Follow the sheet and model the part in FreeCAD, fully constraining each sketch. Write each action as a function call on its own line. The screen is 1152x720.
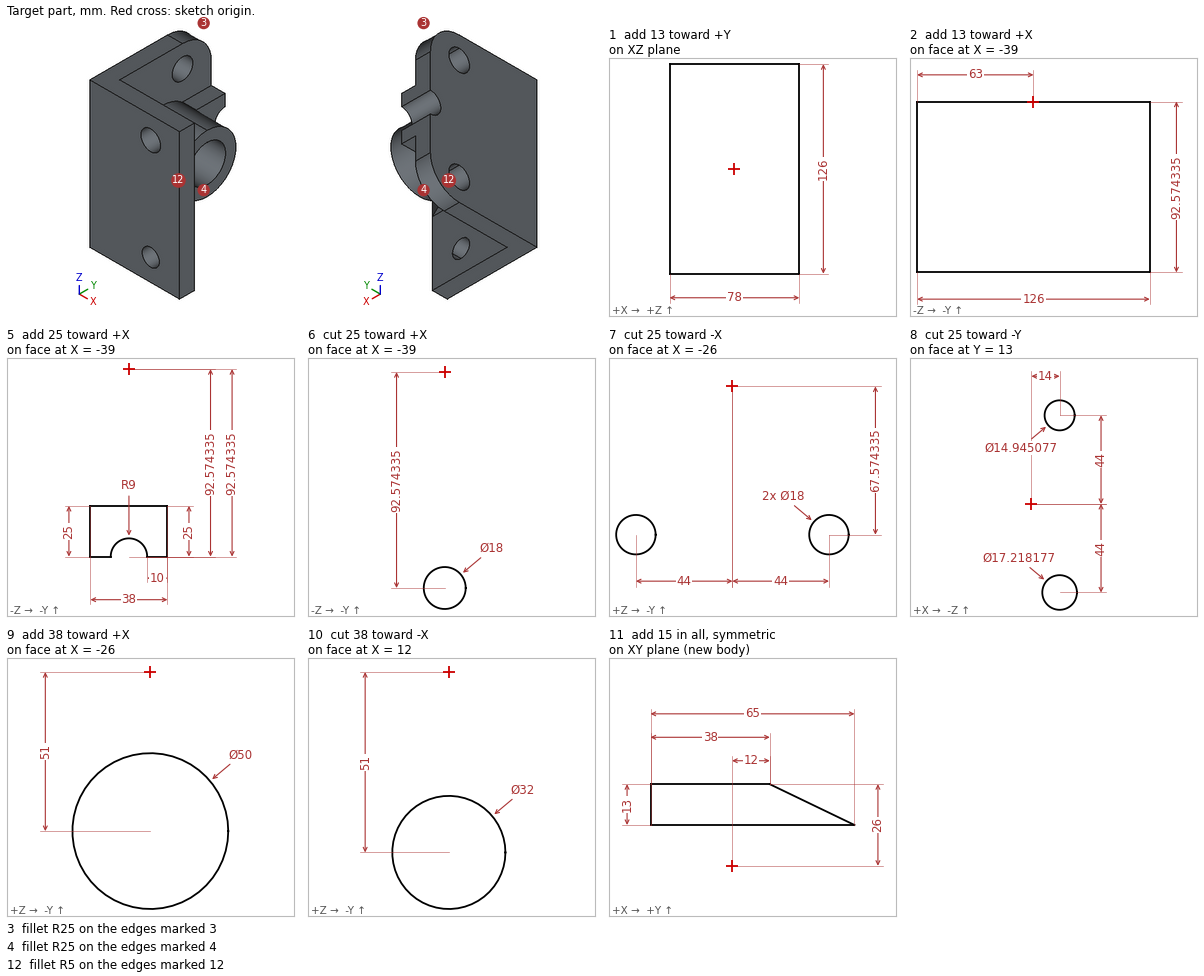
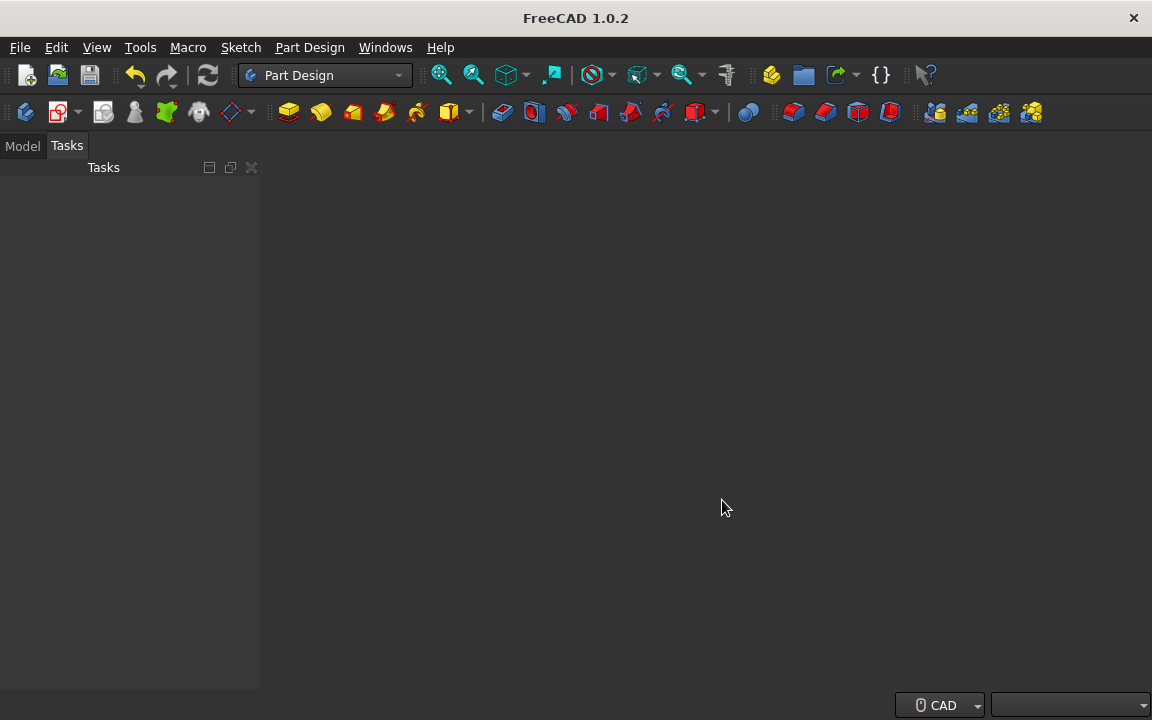
key(ctrl+n)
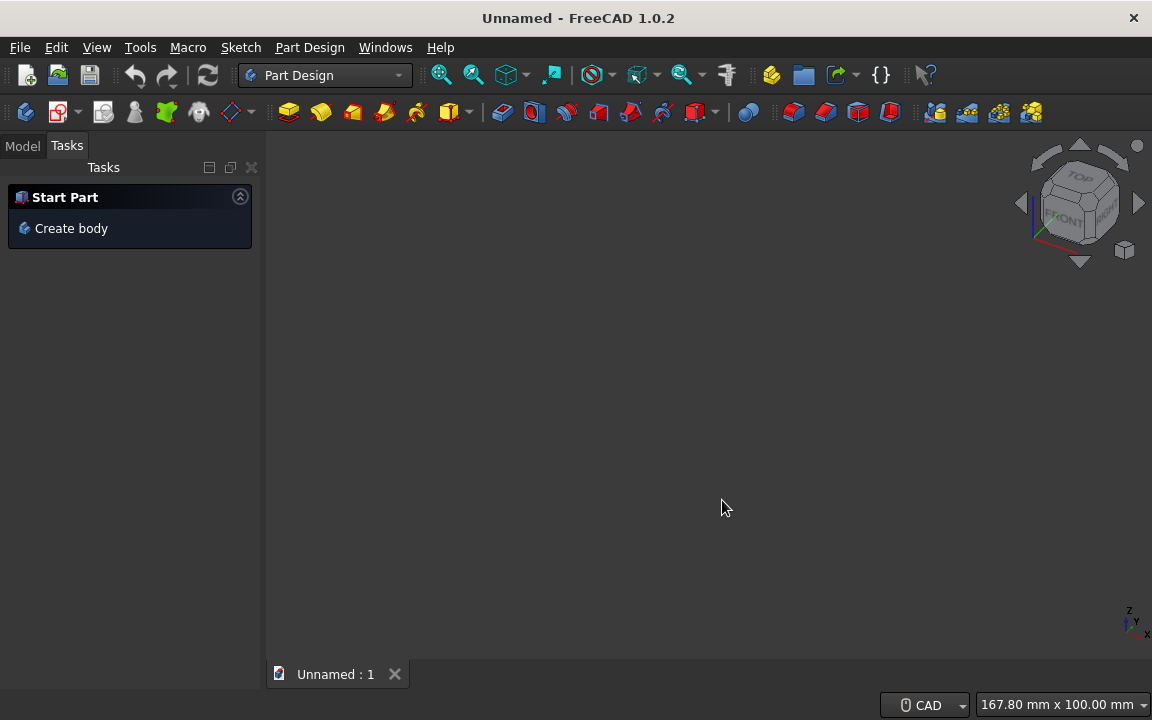
click(58, 112)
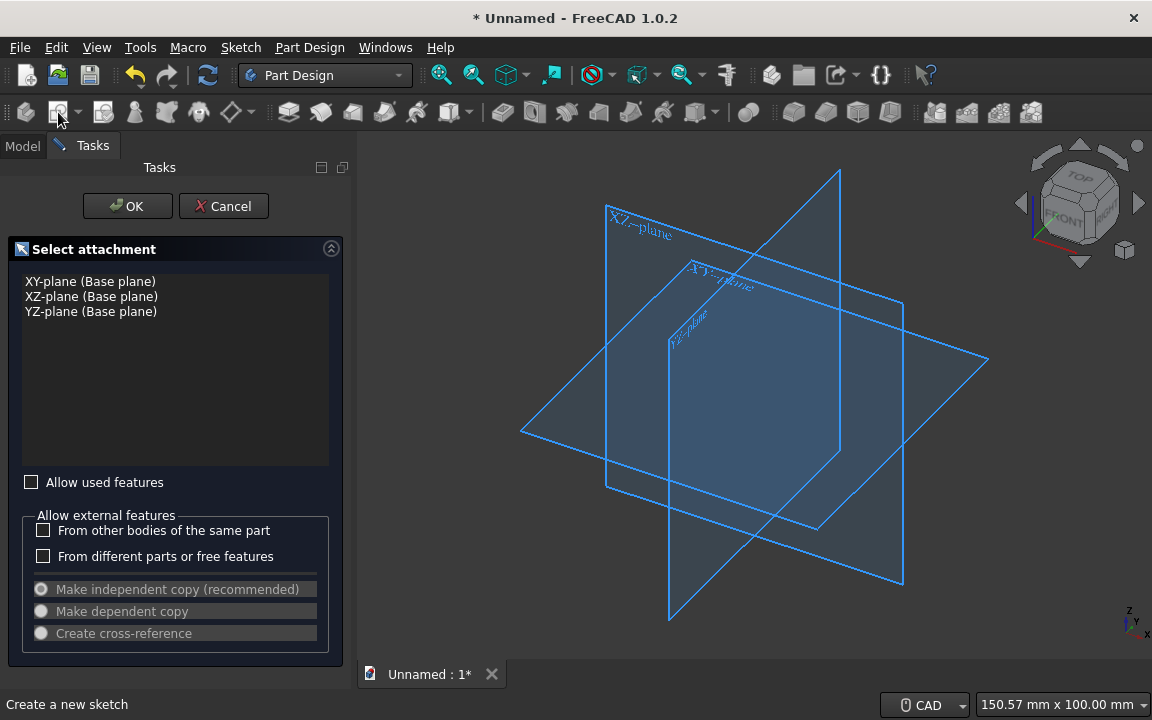
click(82, 296)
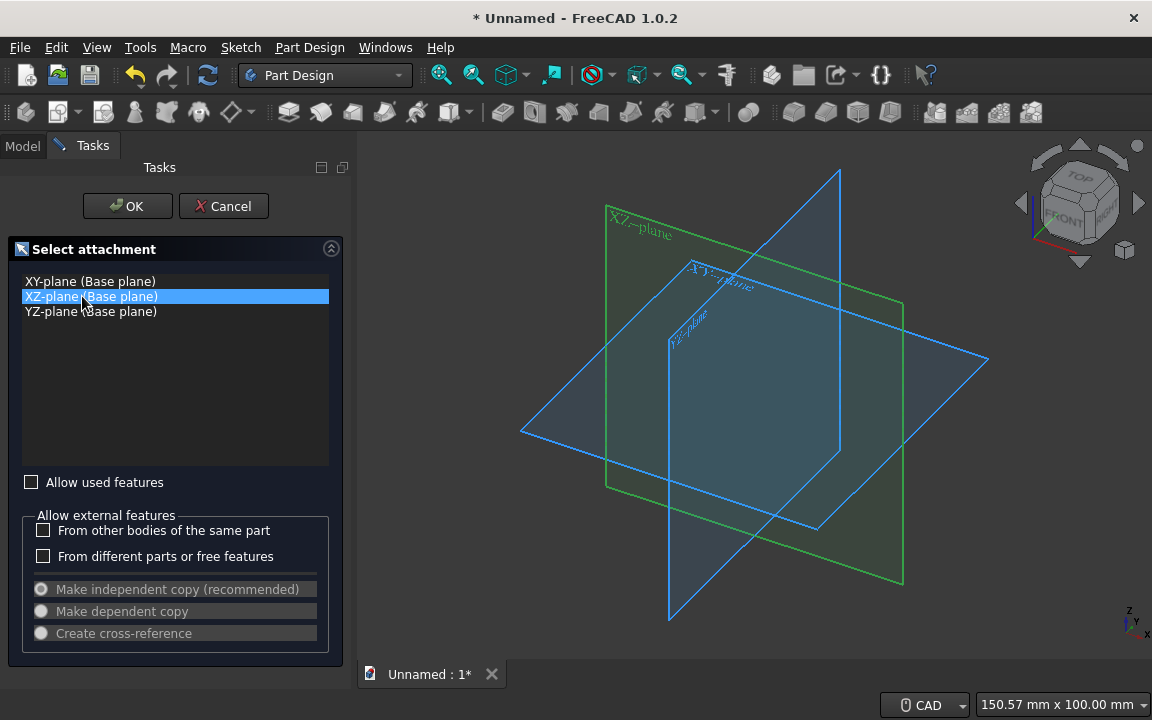
click(128, 206)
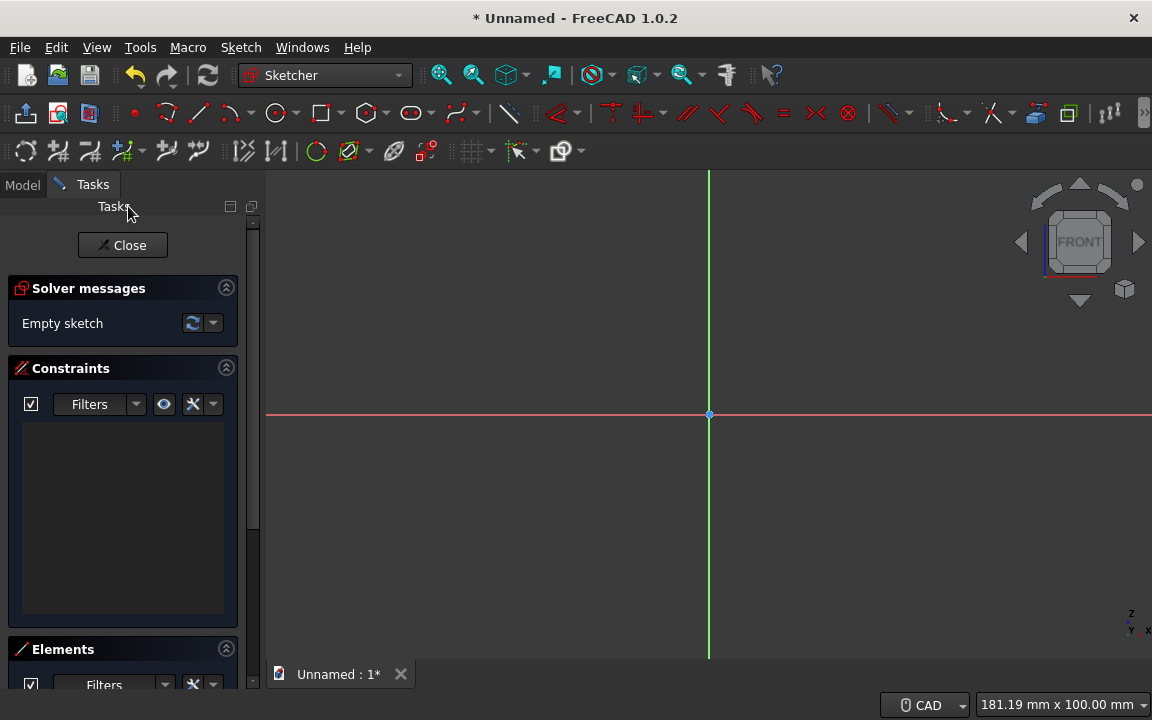
scroll(585, 414, down, 4)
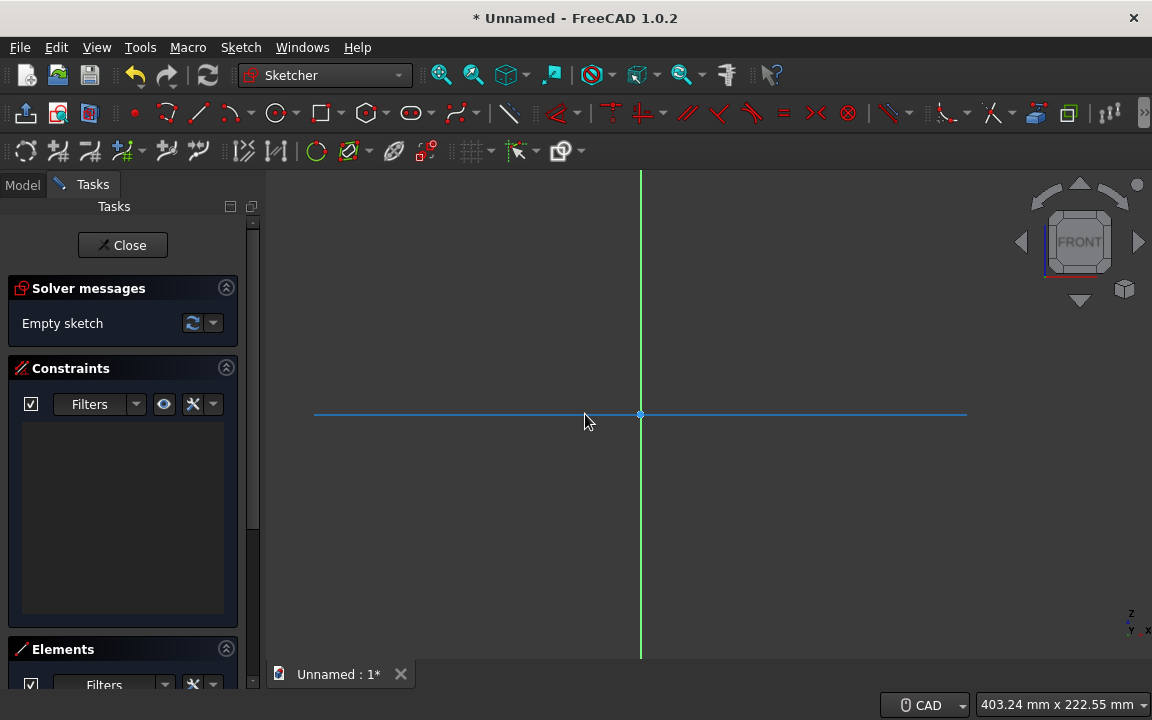
key(g)
key(v)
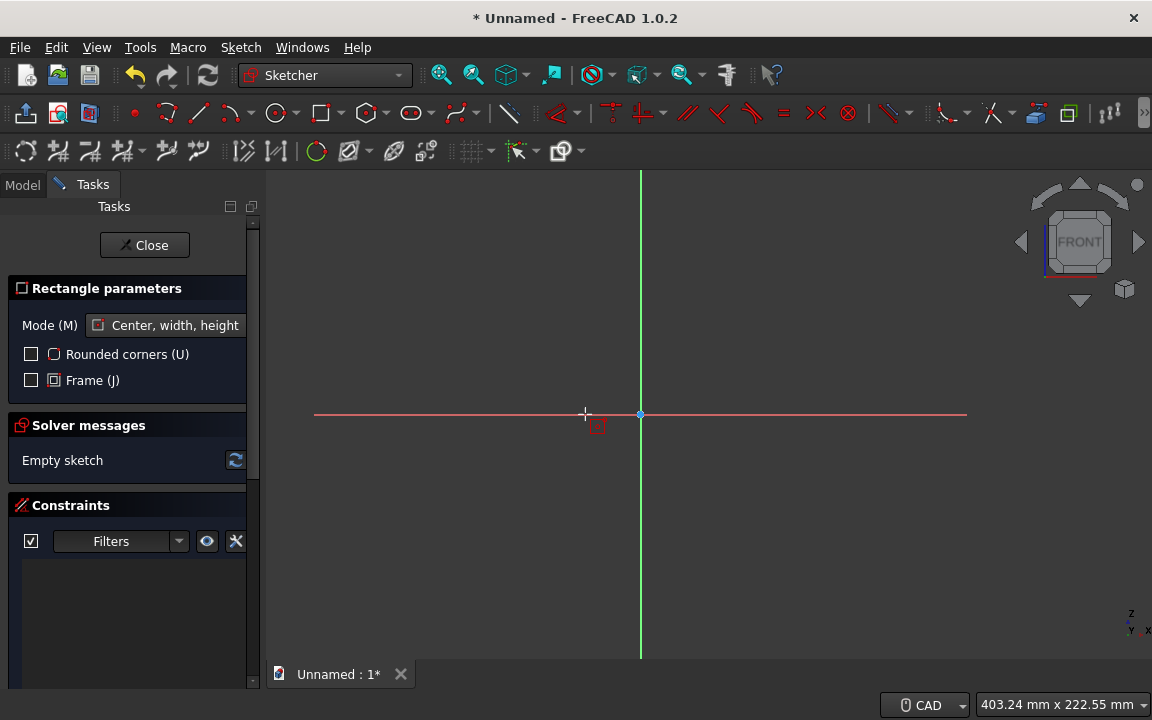
click(641, 414)
move(727, 276)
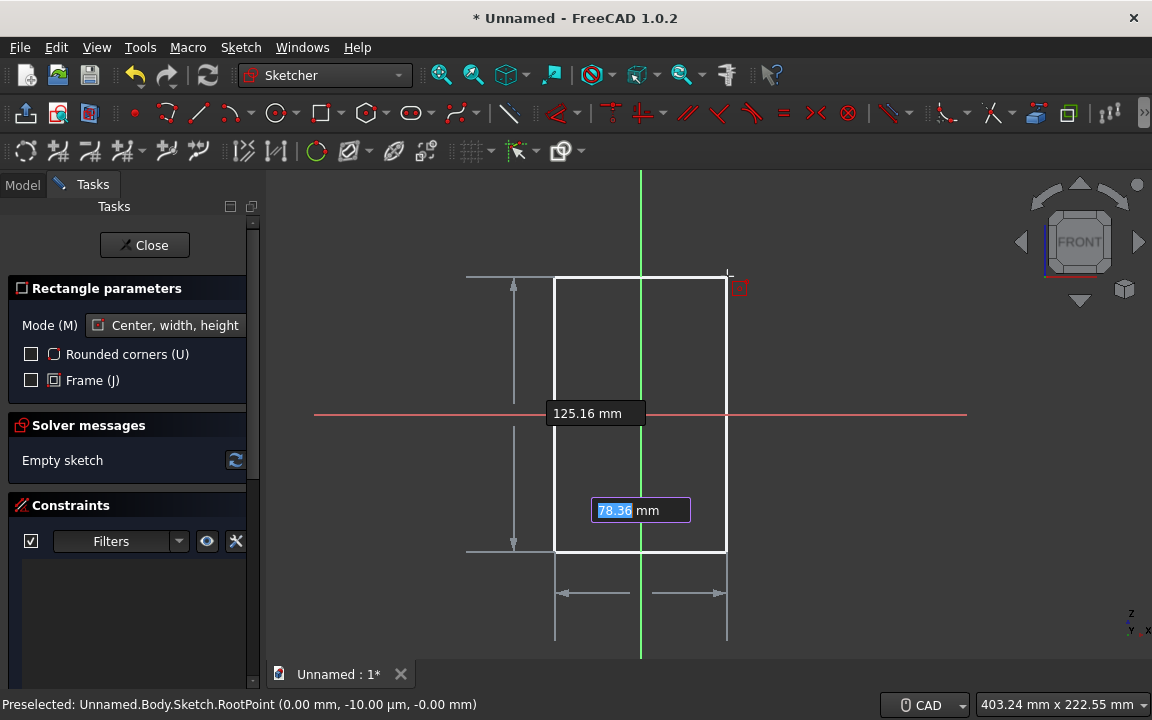
text(78)
key(Tab)
text(126)
key(Return)
key(Escape)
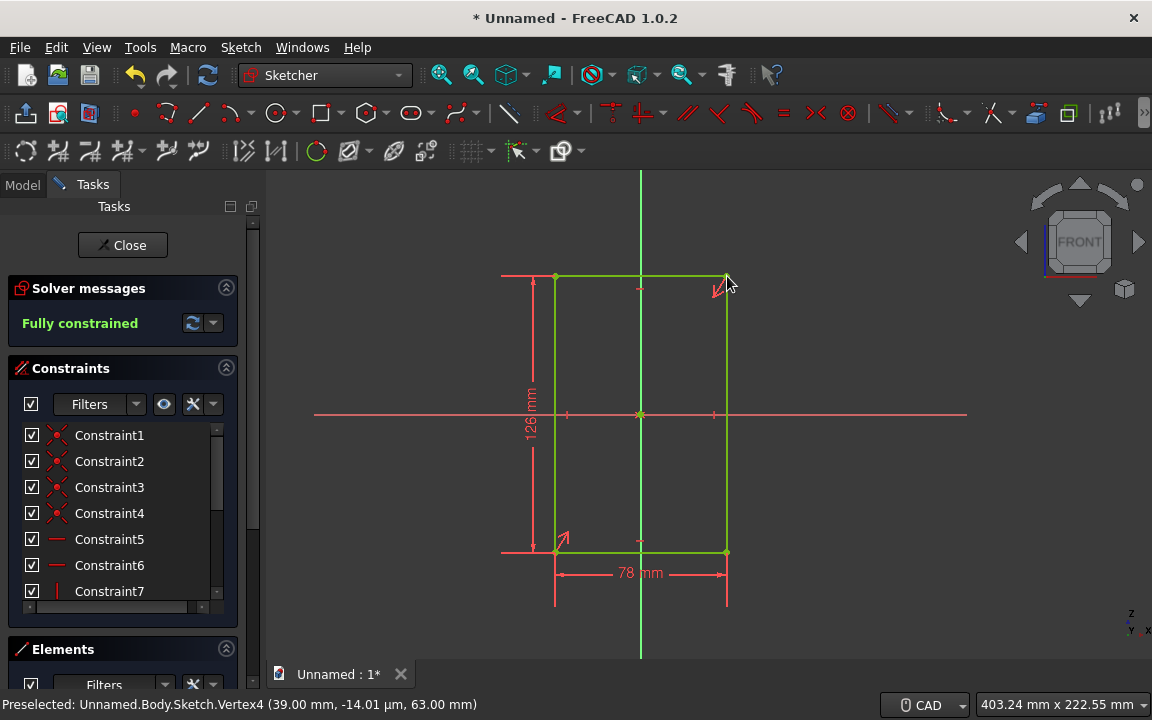
click(123, 245)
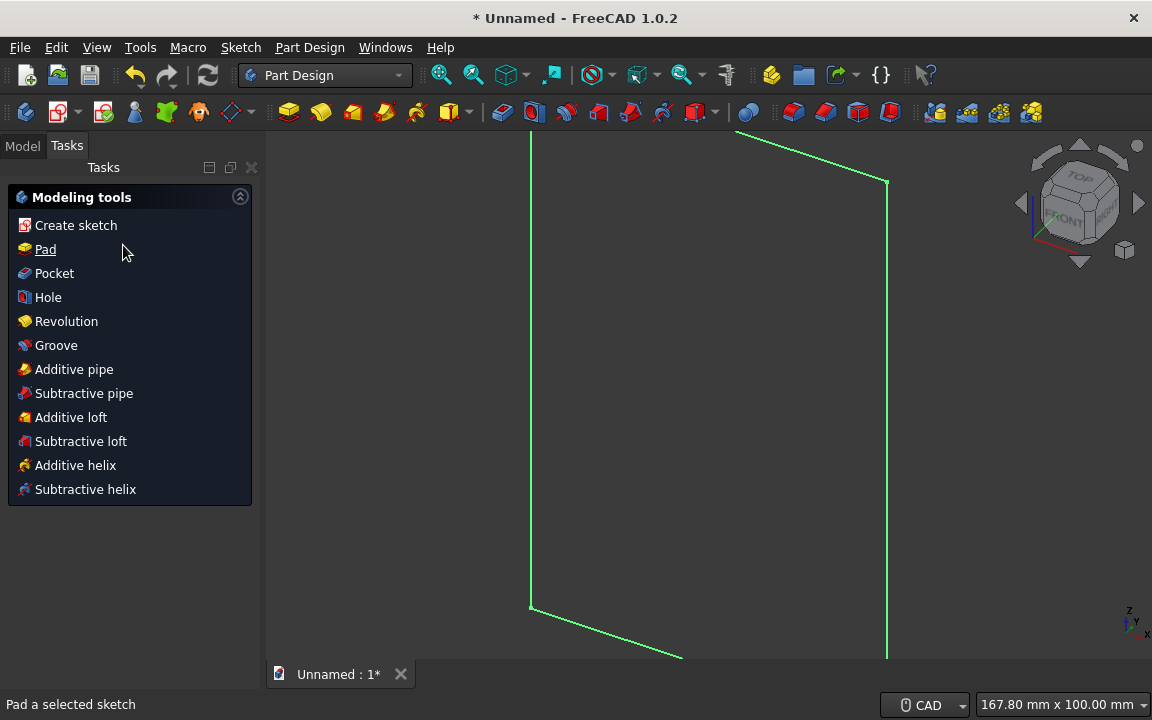
click(290, 112)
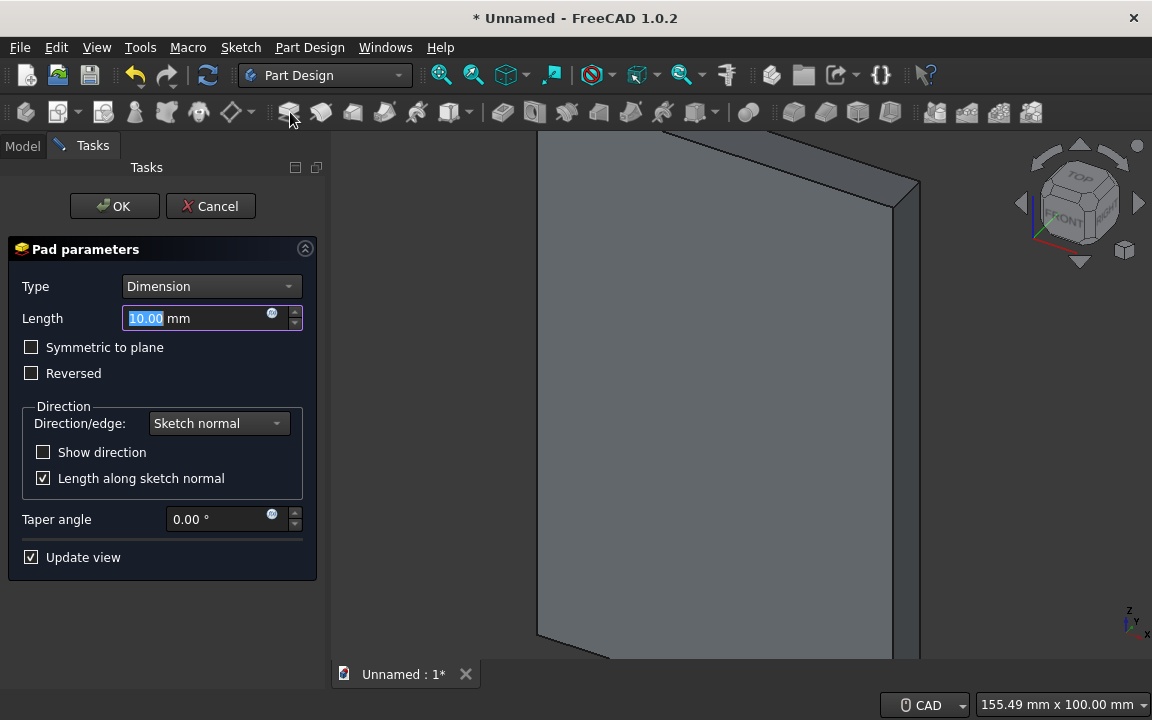
text(13)
key(Tab)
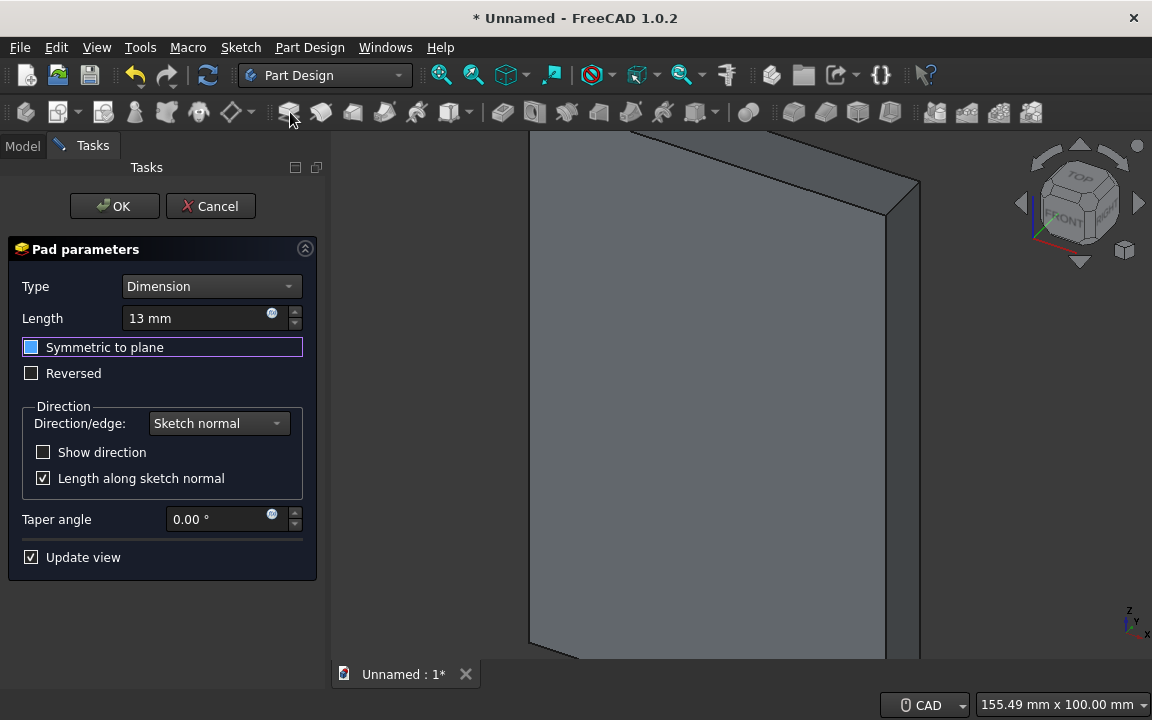
click(30, 373)